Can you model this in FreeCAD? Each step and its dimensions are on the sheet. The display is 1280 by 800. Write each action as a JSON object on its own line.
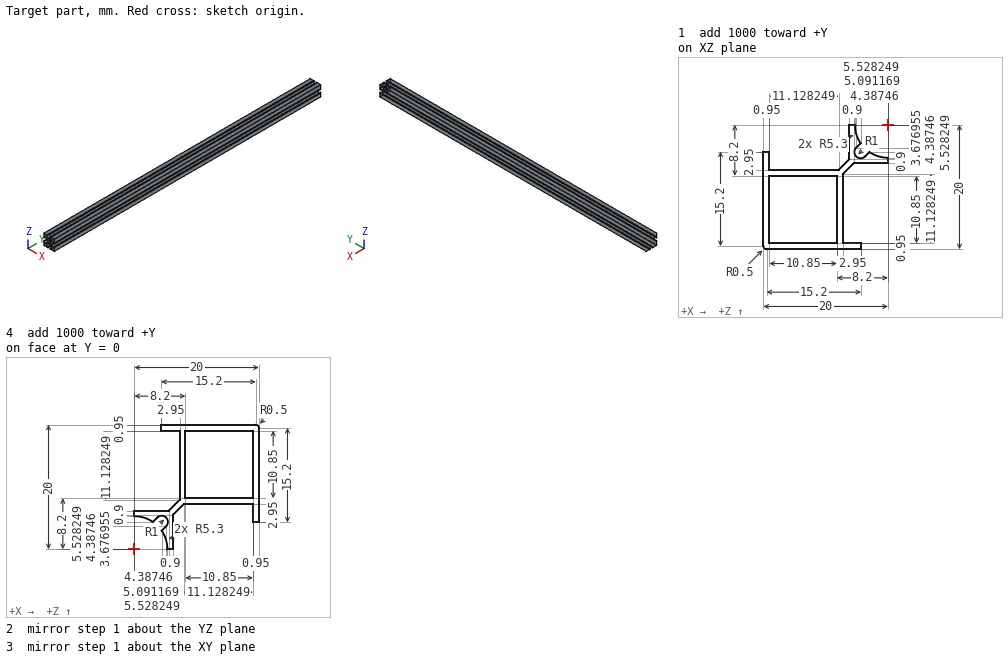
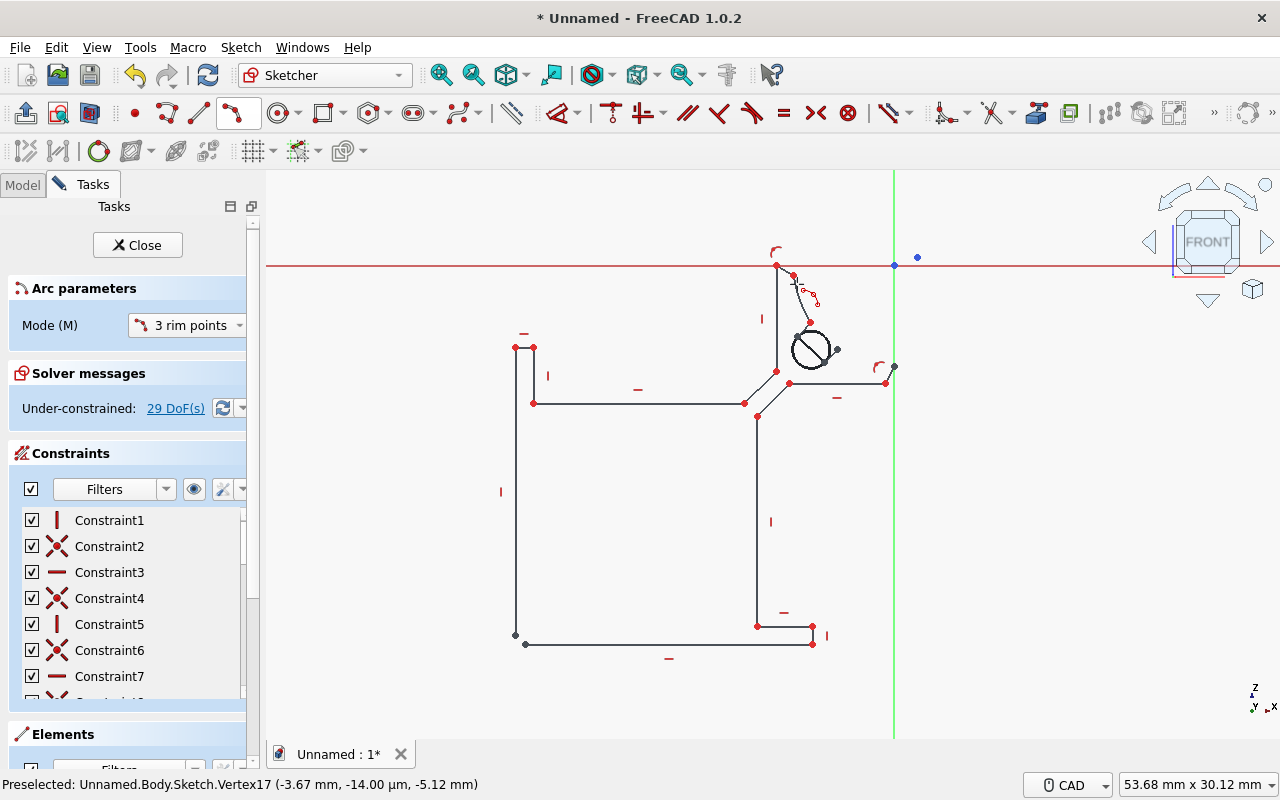
{"action": "left_click", "coordinate": [798, 362]}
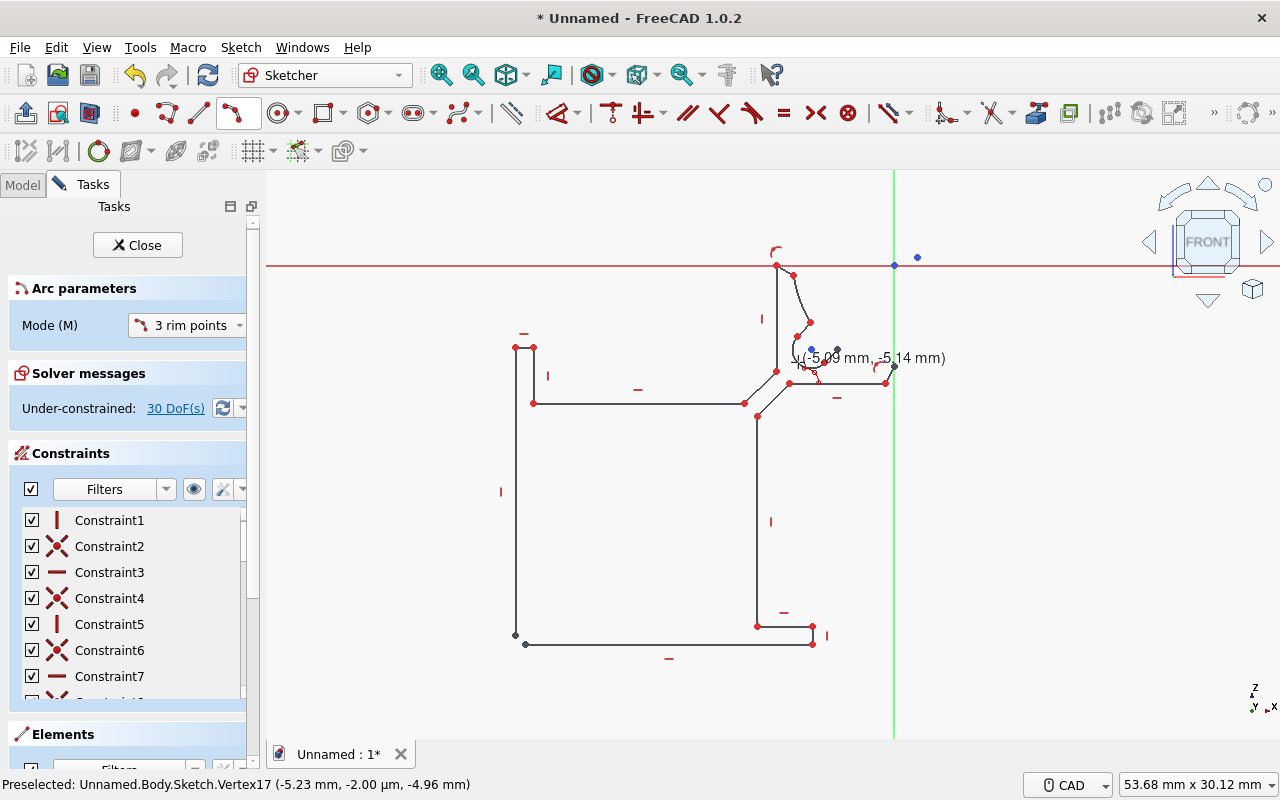
{"action": "scroll", "coordinate": [838, 349], "scroll_direction": "up", "scroll_amount": 3}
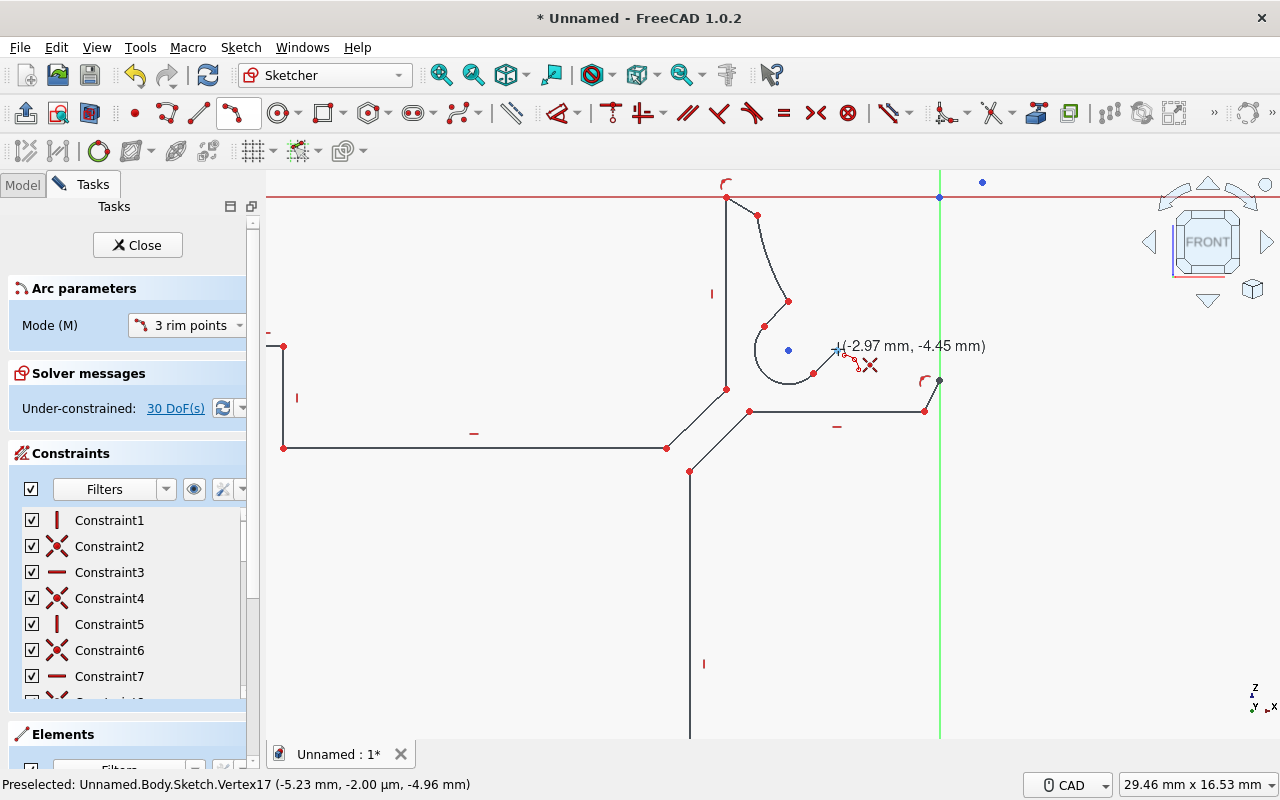
{"action": "left_click", "coordinate": [837, 350]}
{"action": "left_click", "coordinate": [940, 381]}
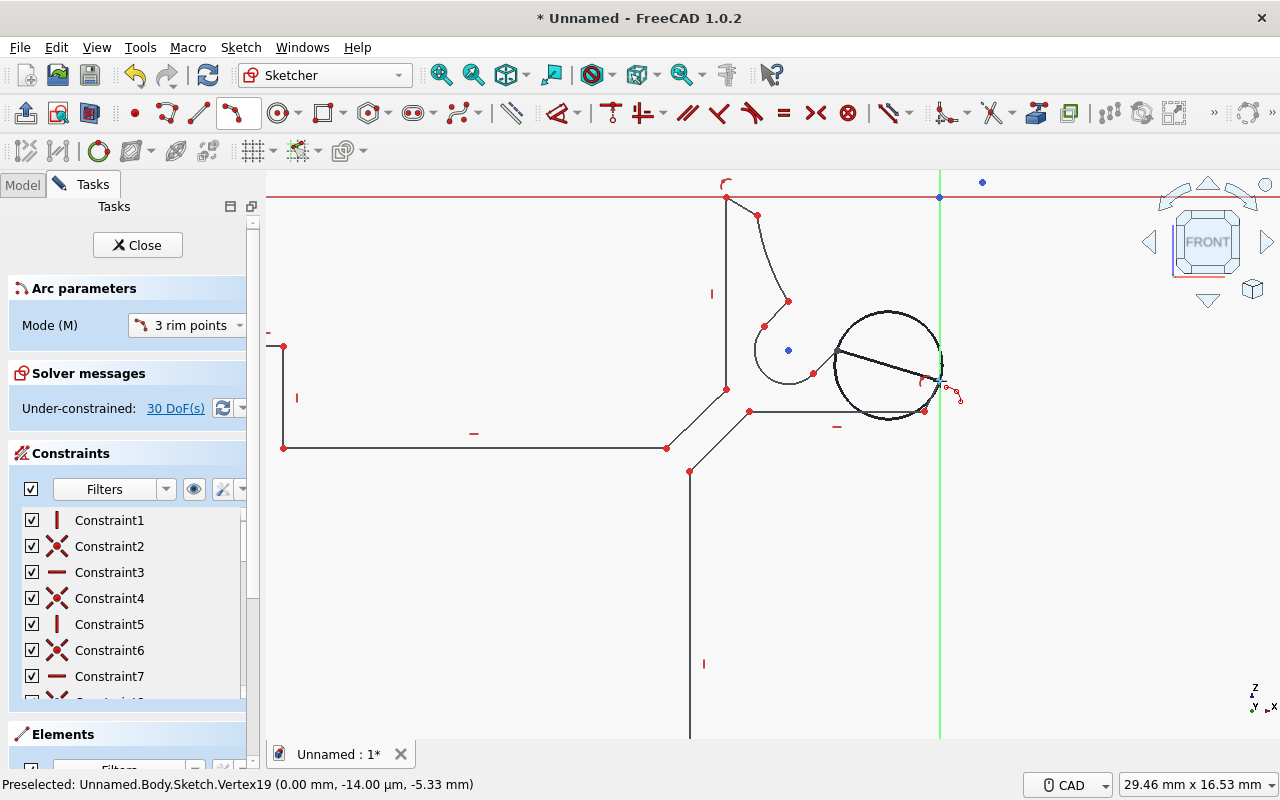
{"action": "scroll", "coordinate": [886, 372], "scroll_direction": "up", "scroll_amount": 4}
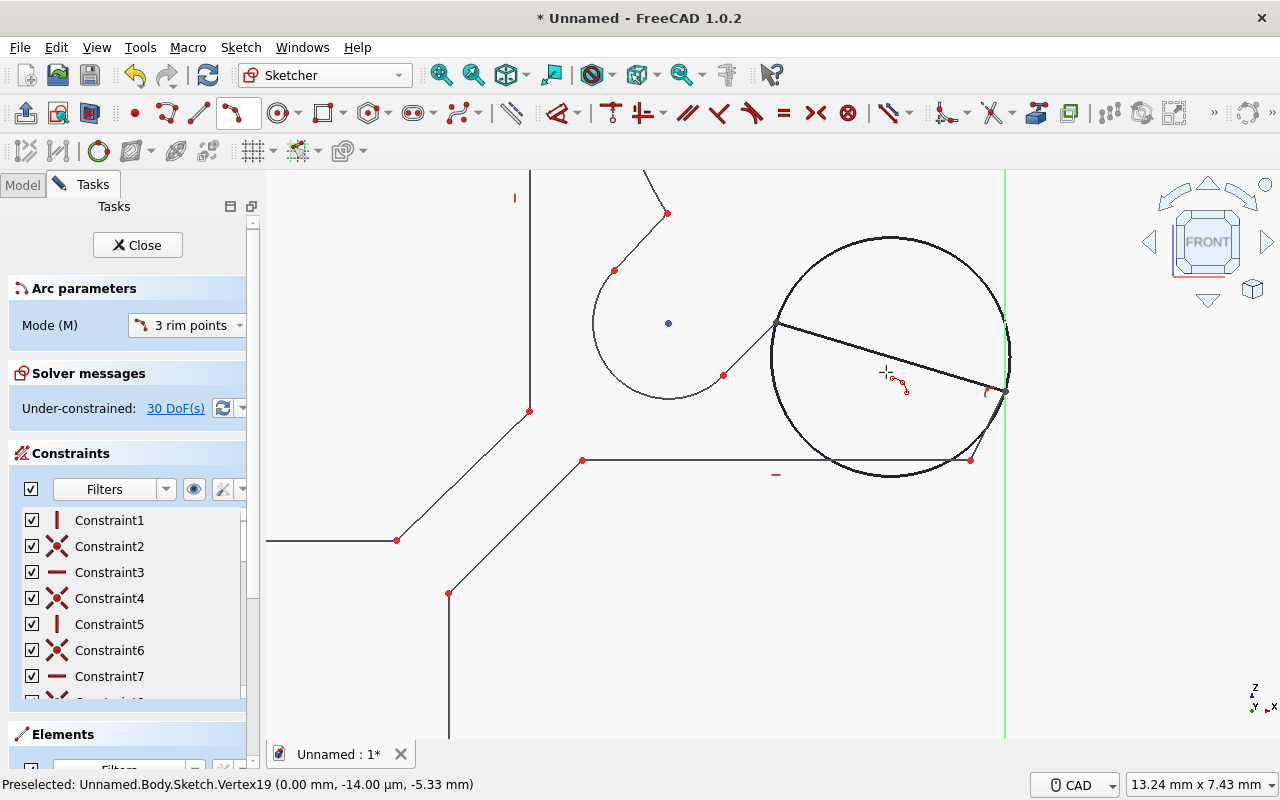
{"action": "left_click", "coordinate": [886, 371]}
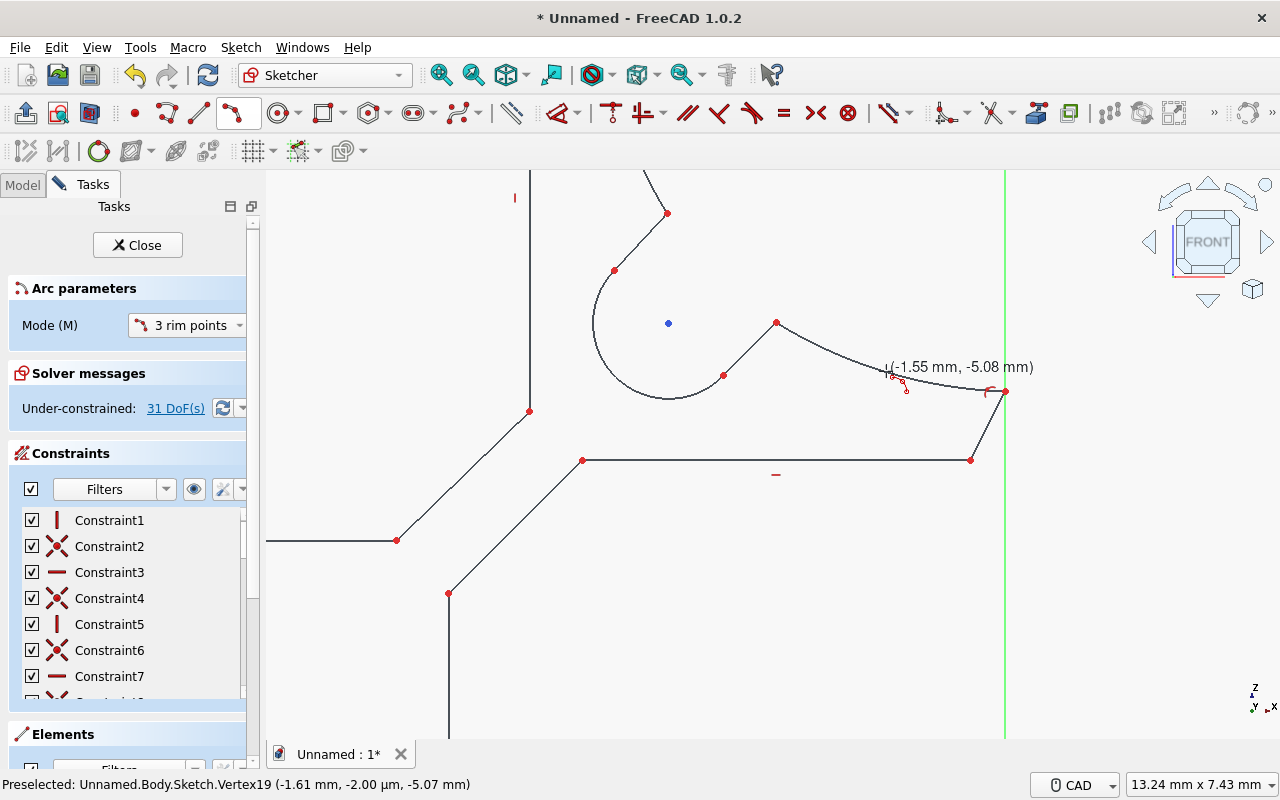
{"action": "scroll", "coordinate": [857, 358], "scroll_direction": "down", "scroll_amount": 7}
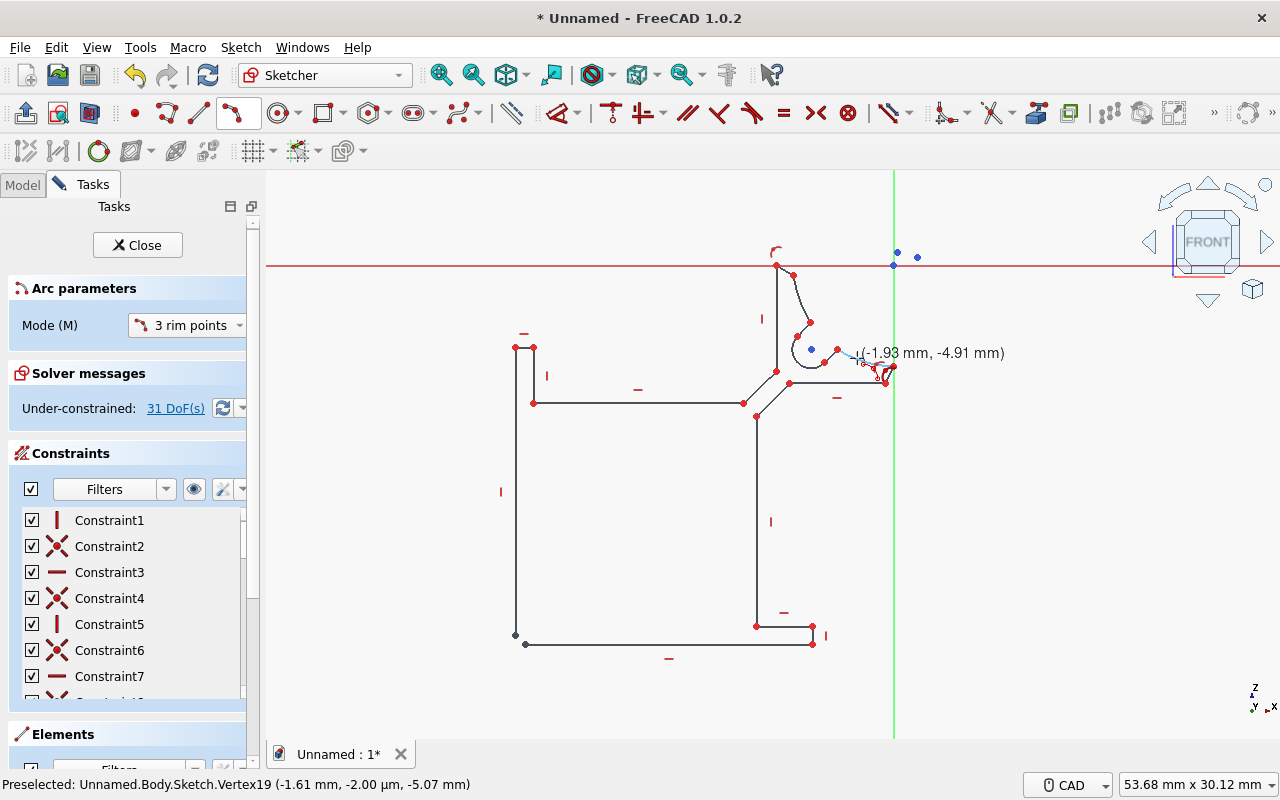
{"action": "left_click", "coordinate": [526, 645]}
{"action": "left_click", "coordinate": [516, 636]}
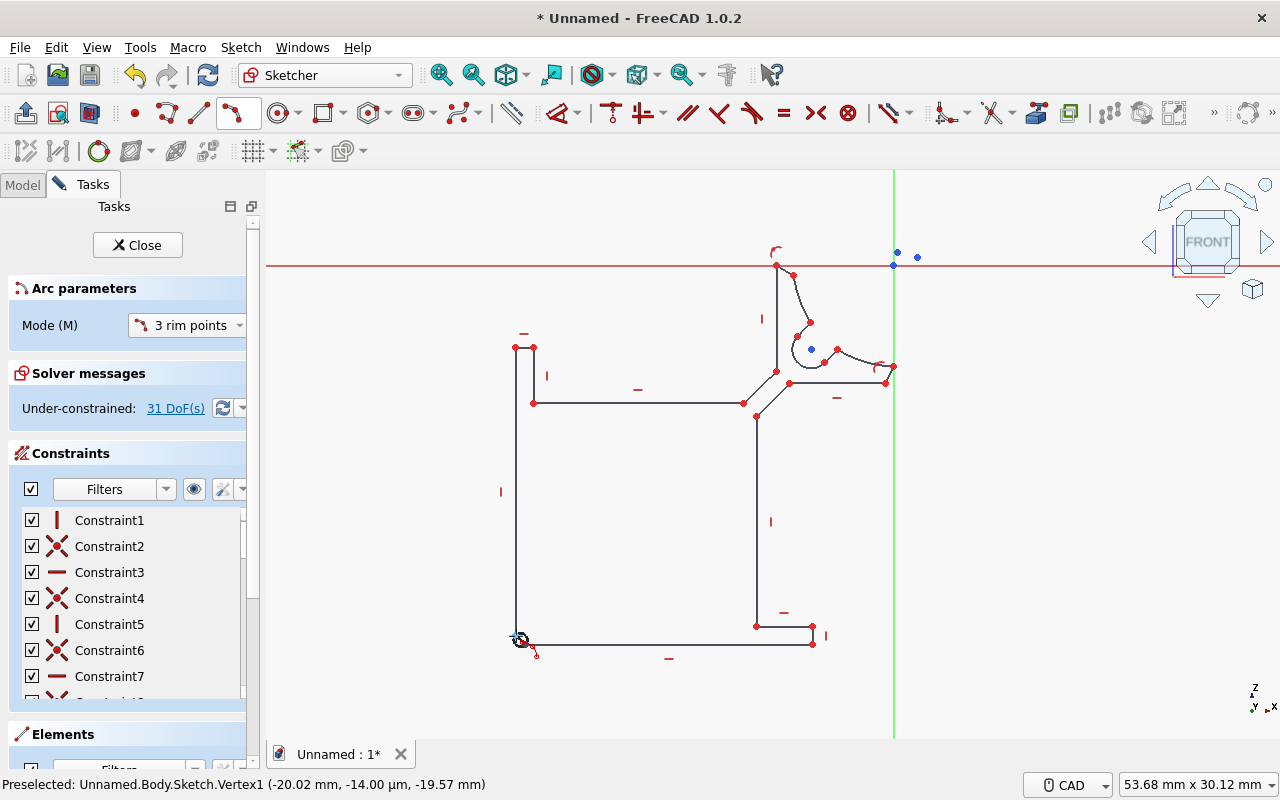
{"action": "scroll", "coordinate": [519, 641], "scroll_direction": "up", "scroll_amount": 9}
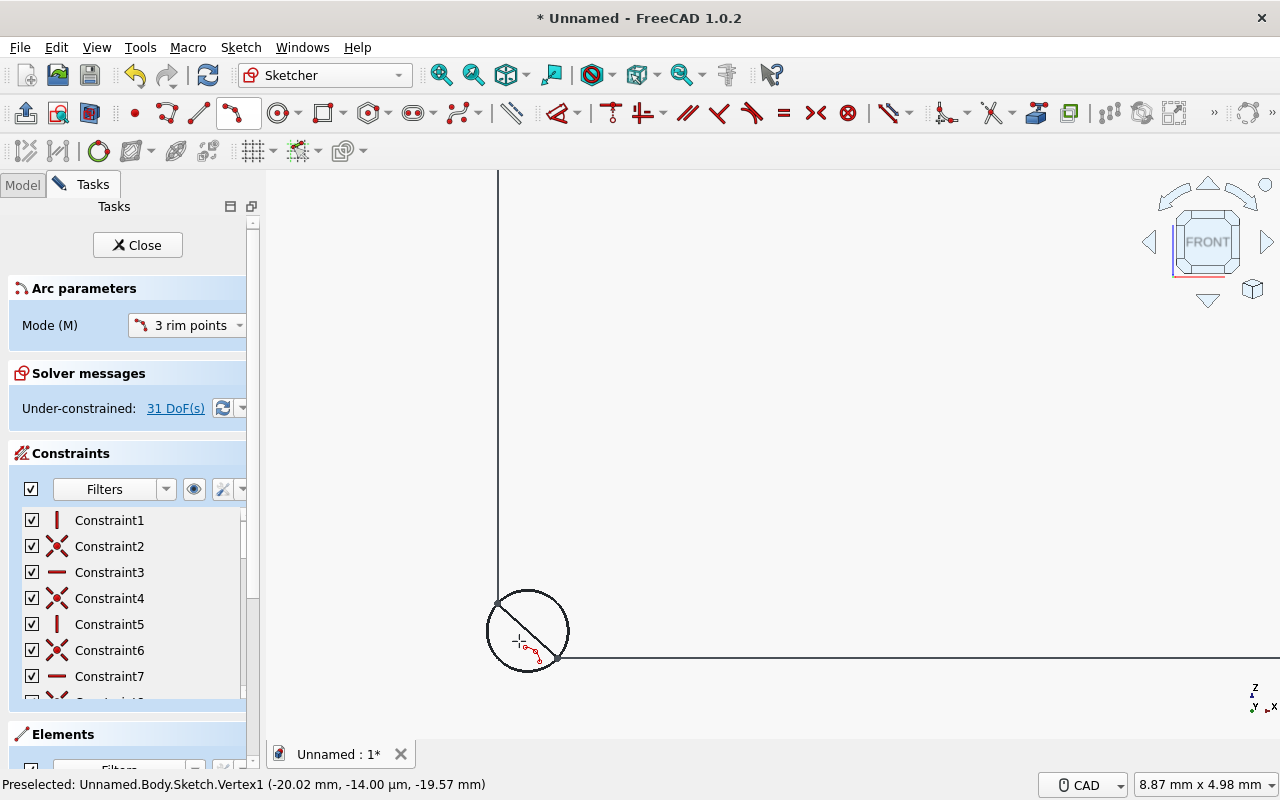
{"action": "left_click", "coordinate": [517, 636]}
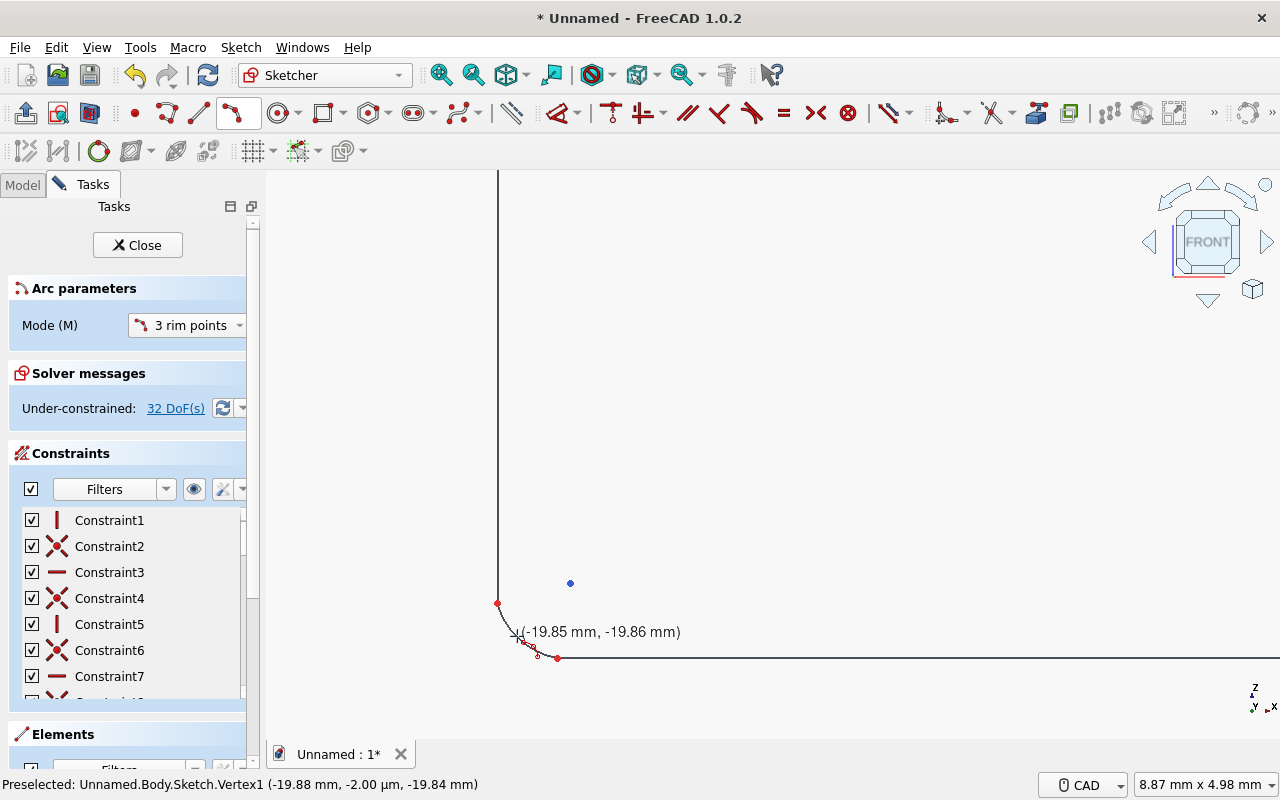
{"action": "left_click", "coordinate": [324, 114]}